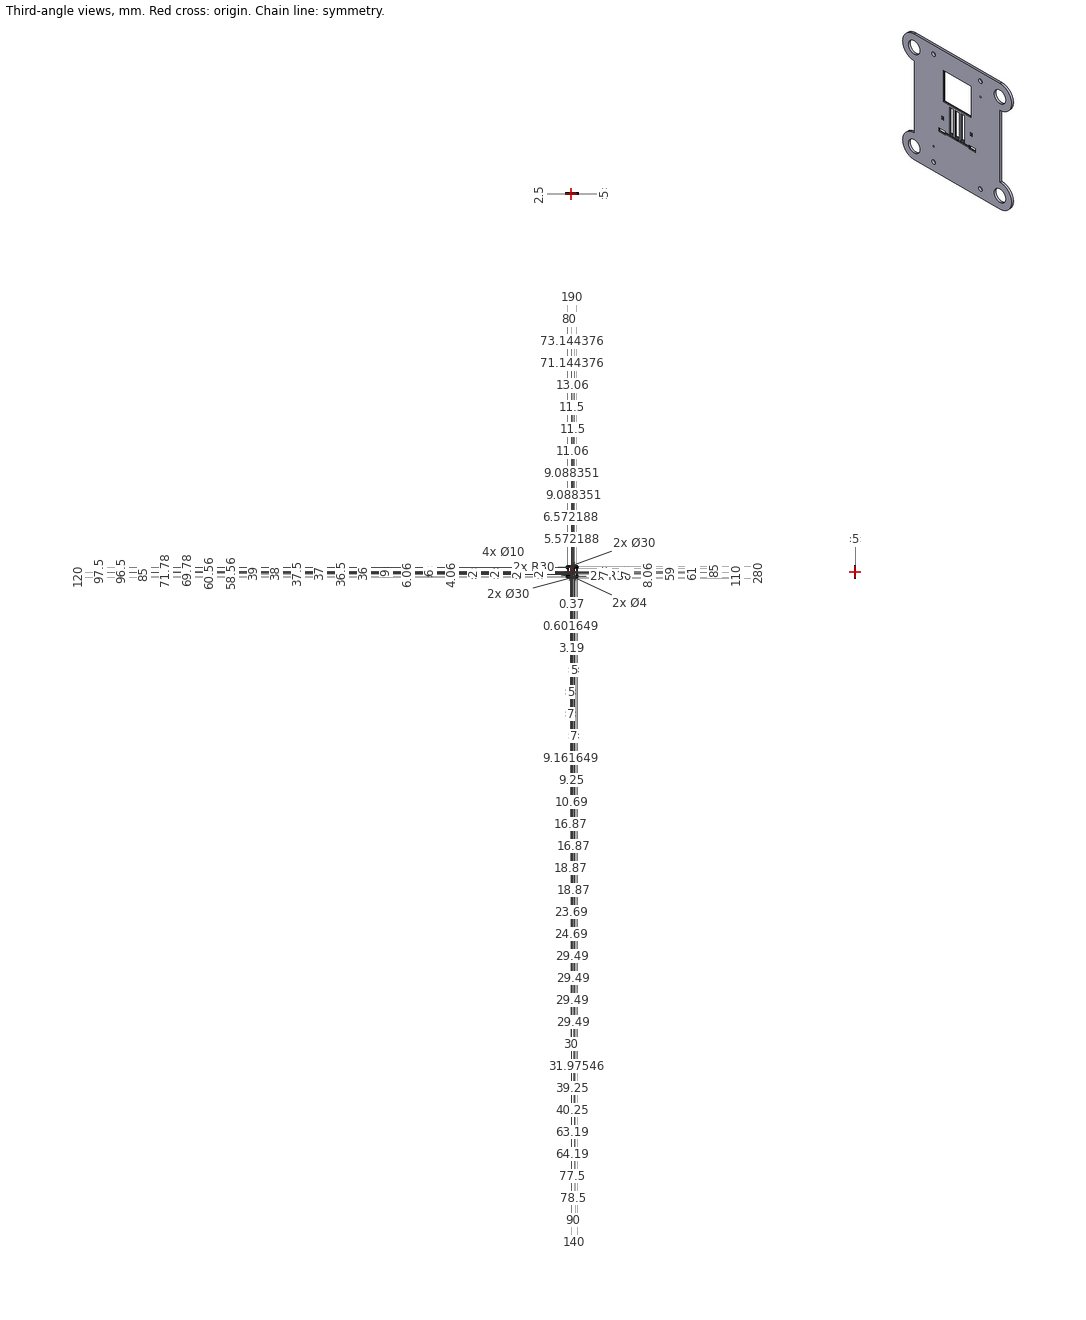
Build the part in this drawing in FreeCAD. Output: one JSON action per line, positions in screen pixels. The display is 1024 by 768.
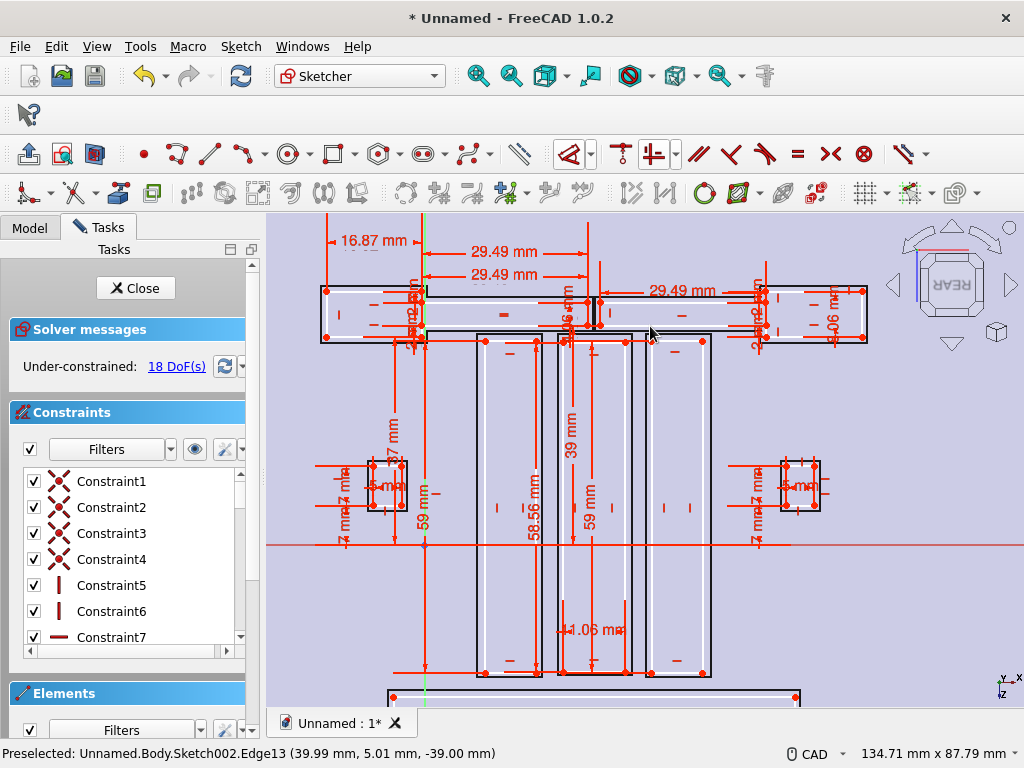
{"action": "left_click", "coordinate": [795, 337]}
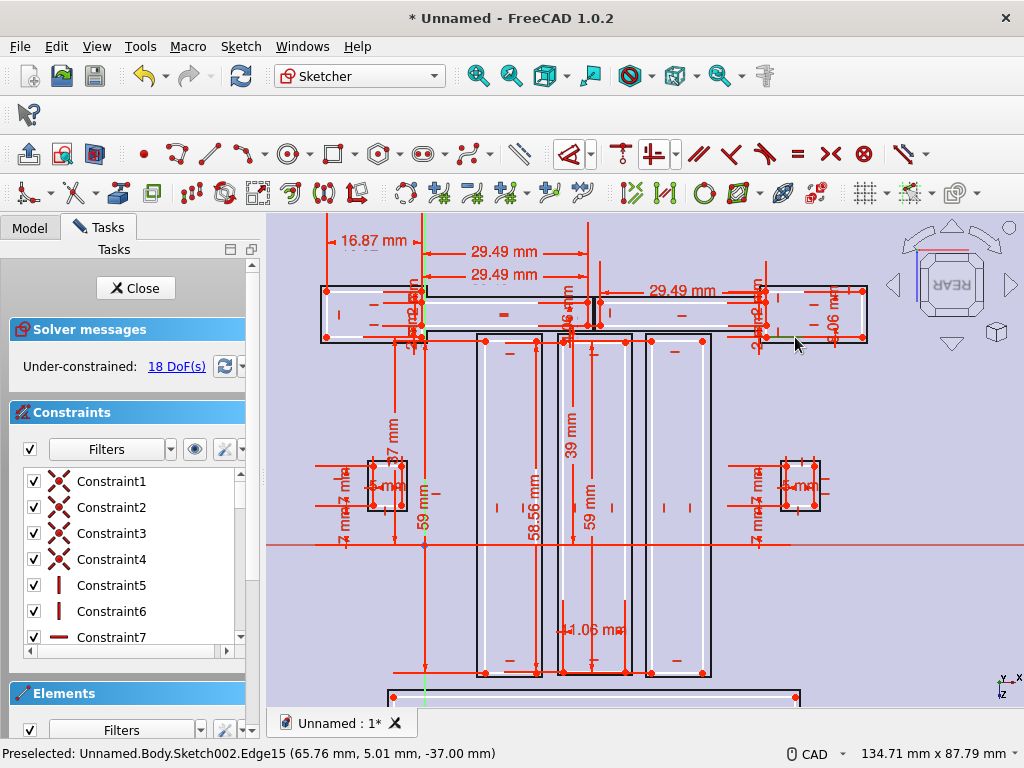
{"action": "key", "text": "l"}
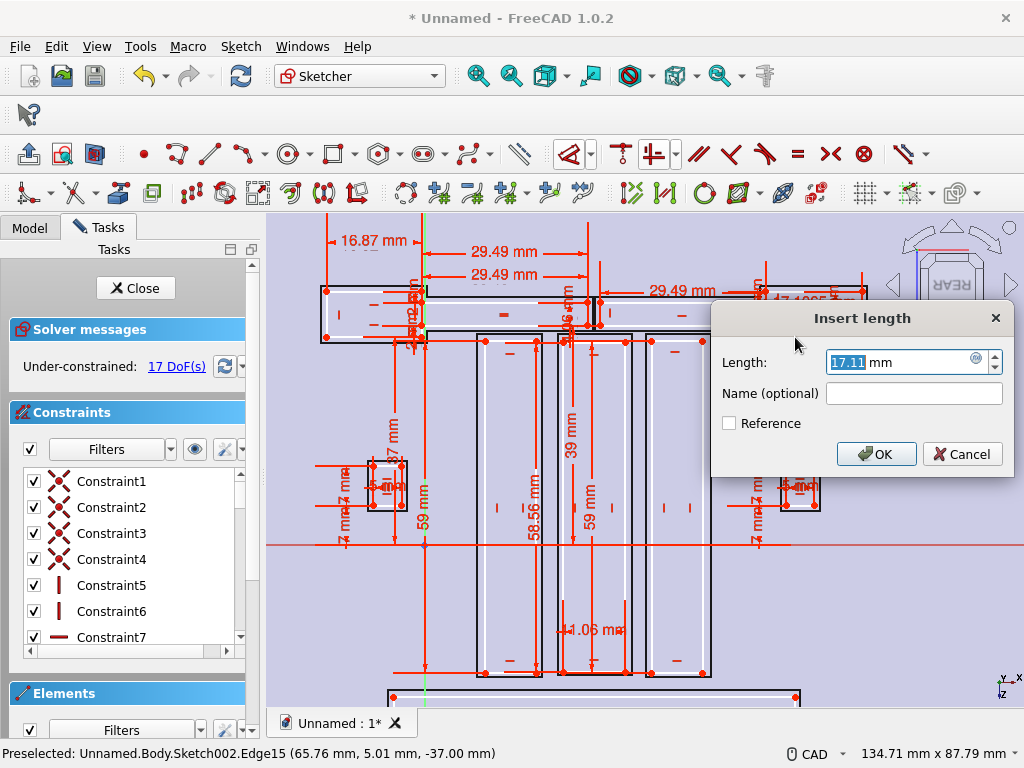
{"action": "type", "text": "16.87"}
{"action": "key", "text": "Return"}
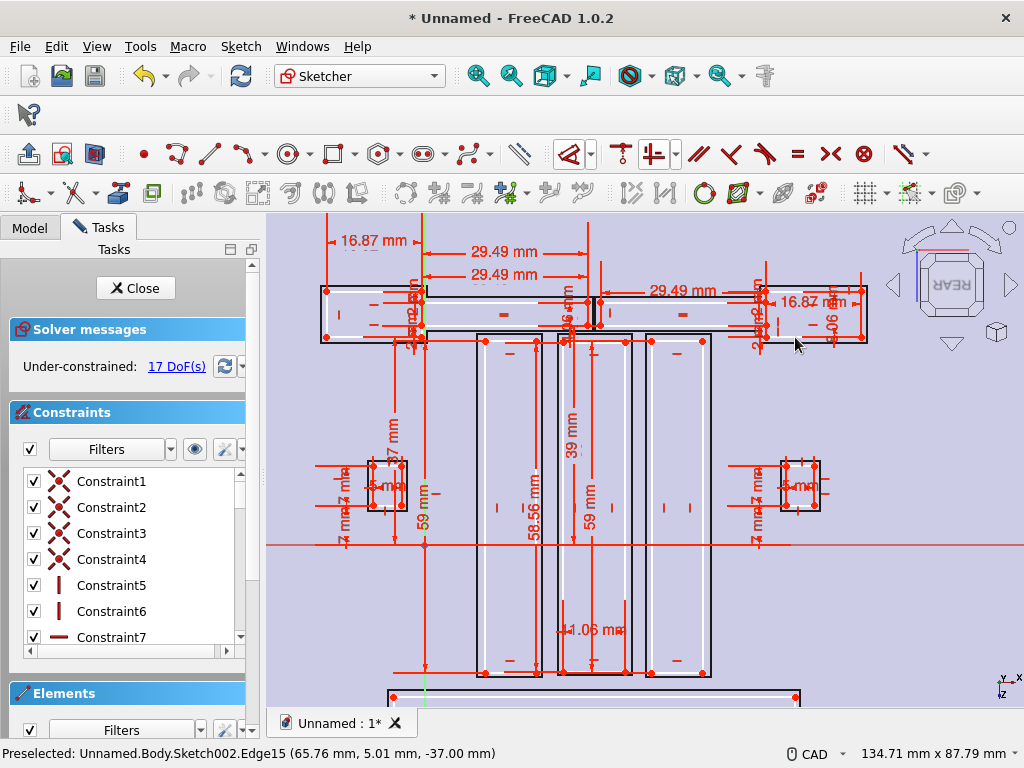
{"action": "left_click", "coordinate": [795, 292]}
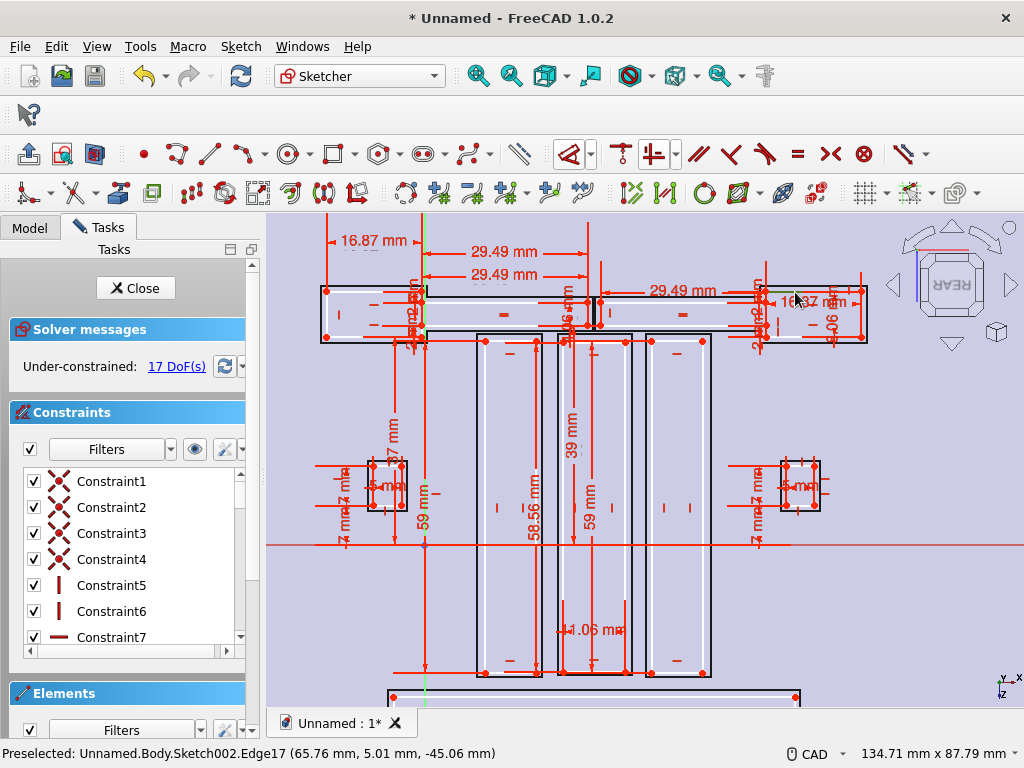
{"action": "key", "text": "l"}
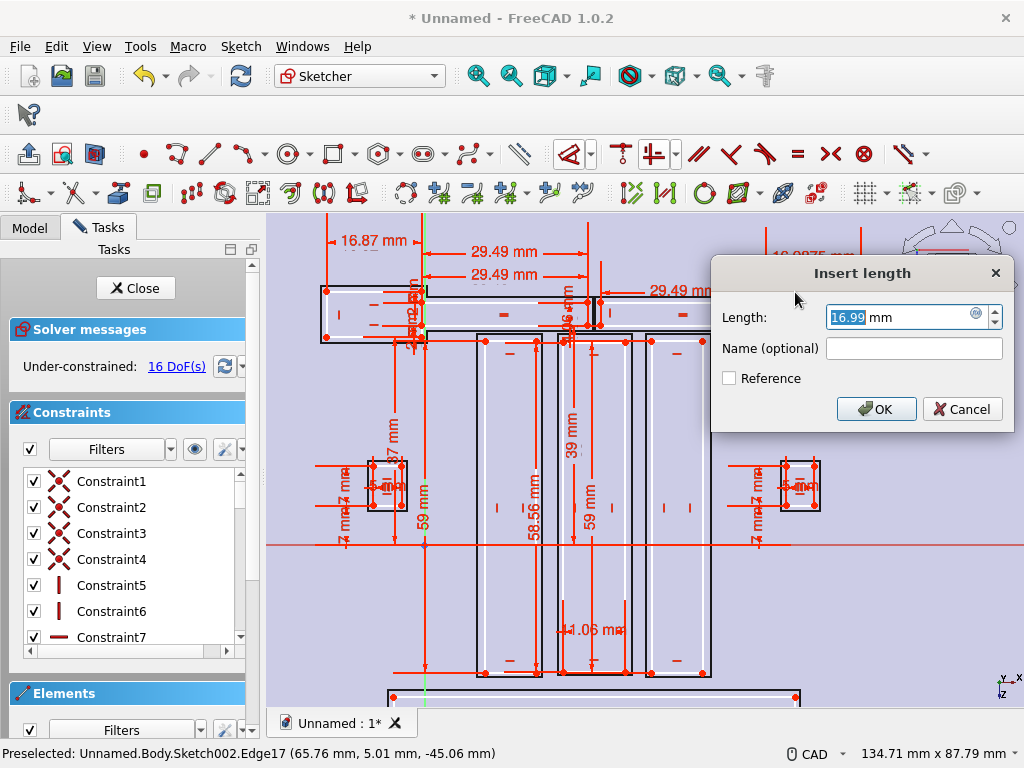
{"action": "type", "text": "16.87"}
{"action": "key", "text": "Return"}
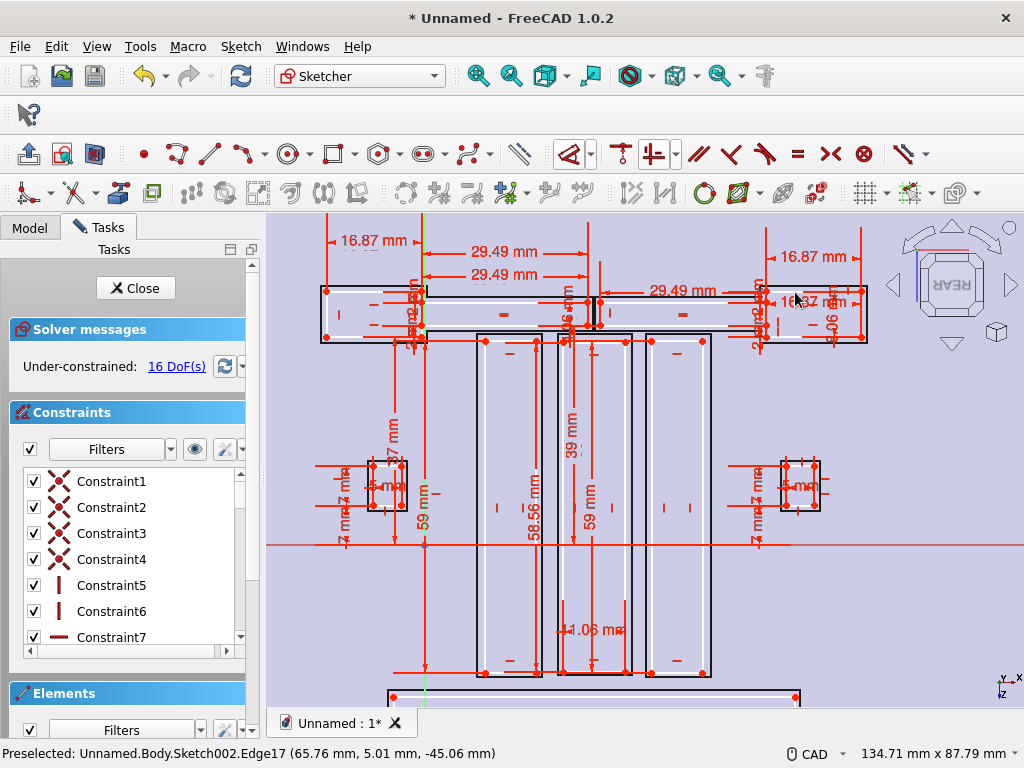
{"action": "scroll", "coordinate": [566, 326], "scroll_direction": "down", "scroll_amount": 5}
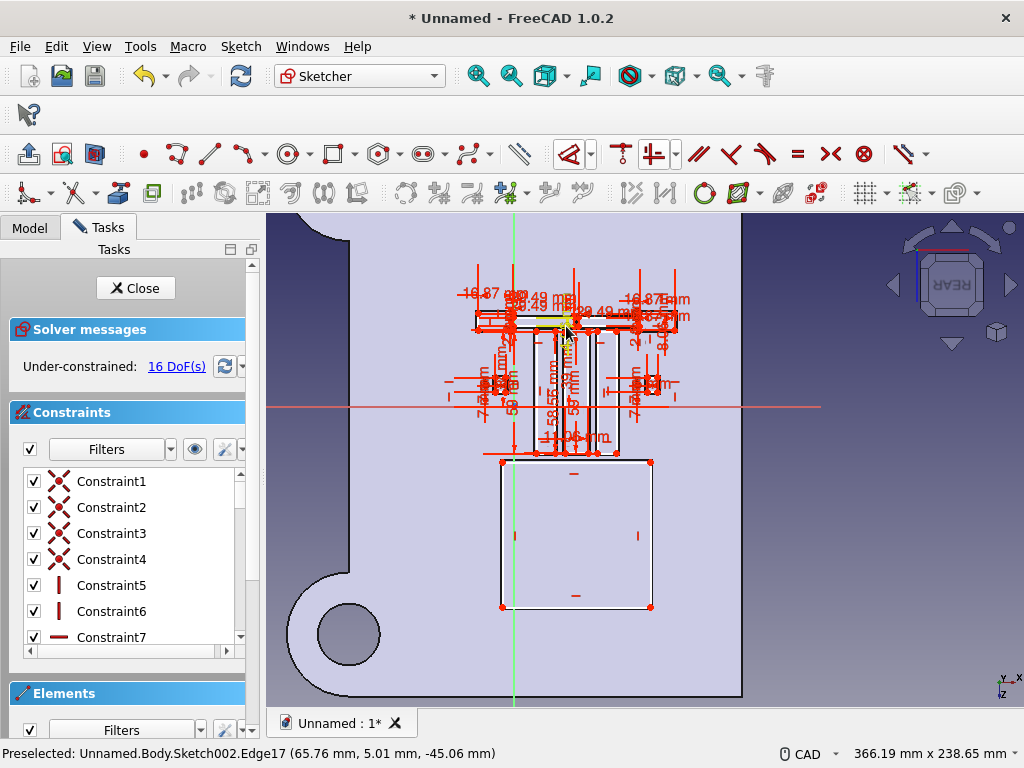
{"action": "left_click", "coordinate": [503, 506]}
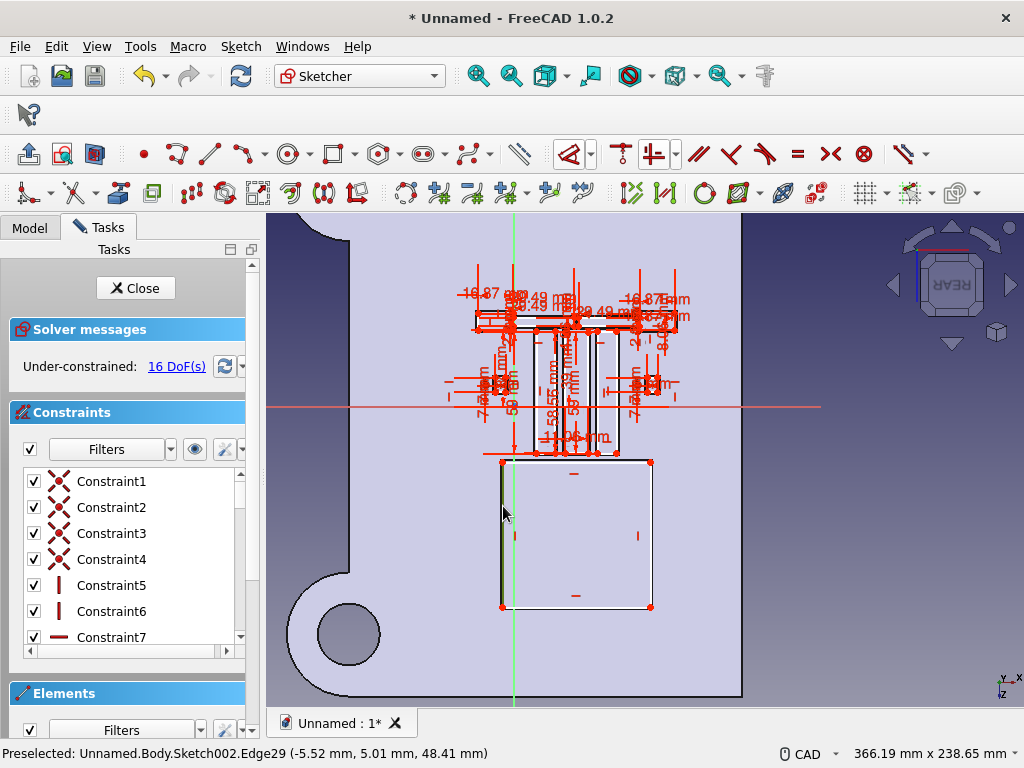
{"action": "left_click", "coordinate": [590, 154]}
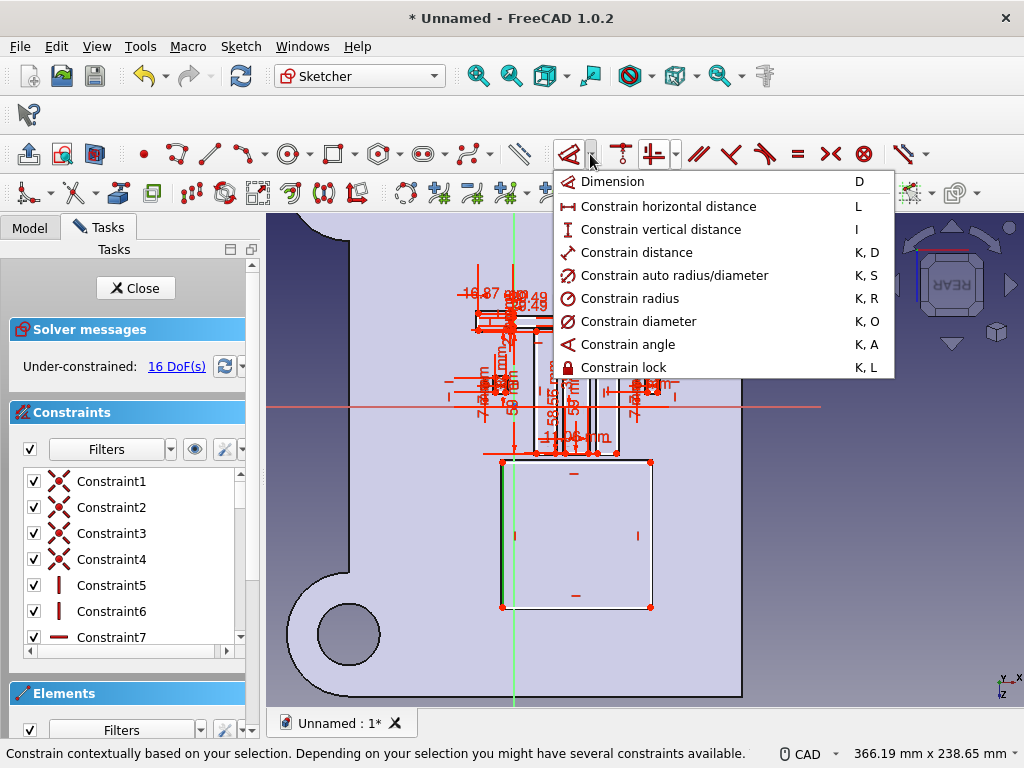
{"action": "left_click", "coordinate": [724, 230]}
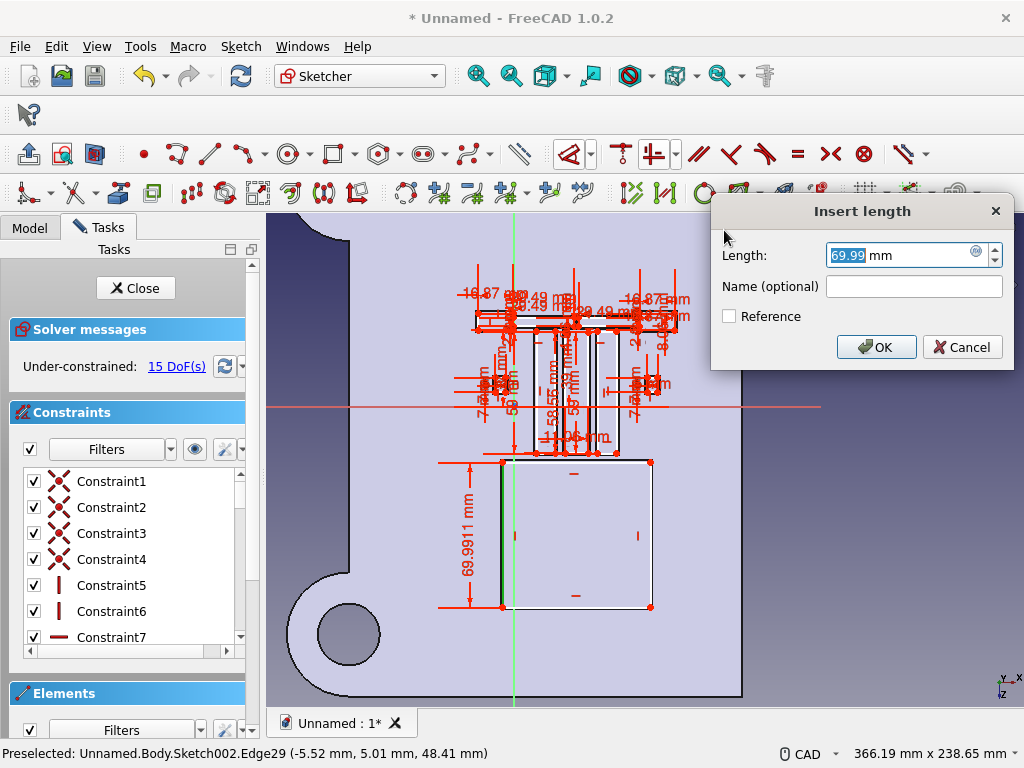
{"action": "type", "text": "69.78"}
{"action": "key", "text": "Return"}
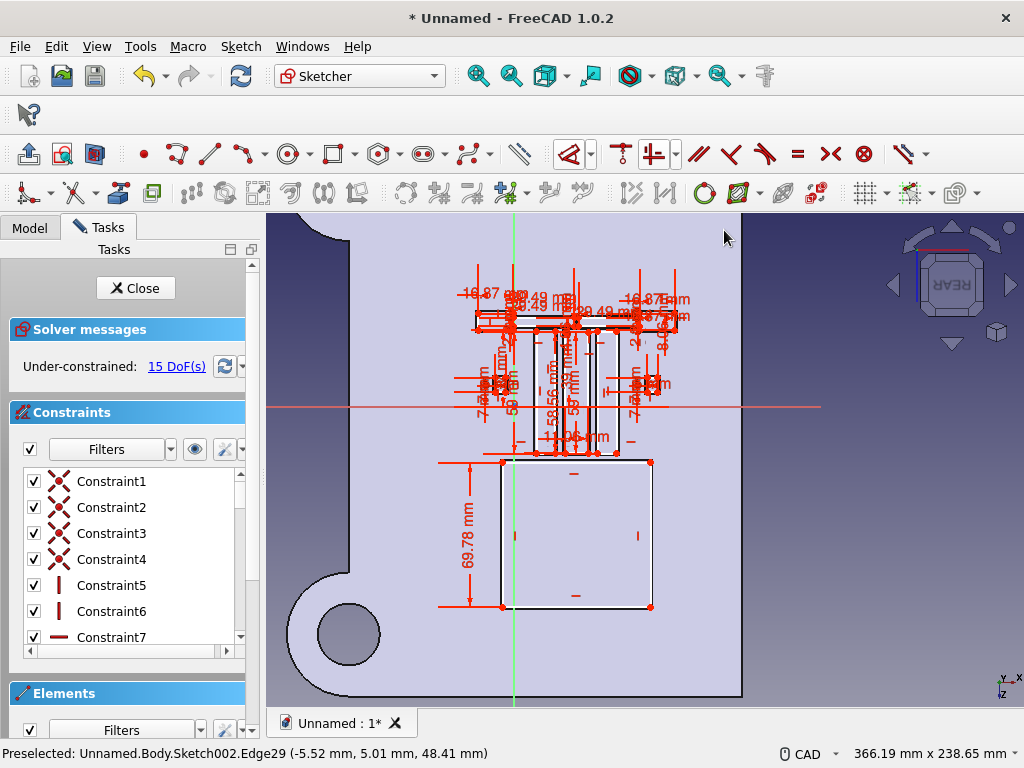
{"action": "scroll", "coordinate": [565, 332], "scroll_direction": "up", "scroll_amount": 2}